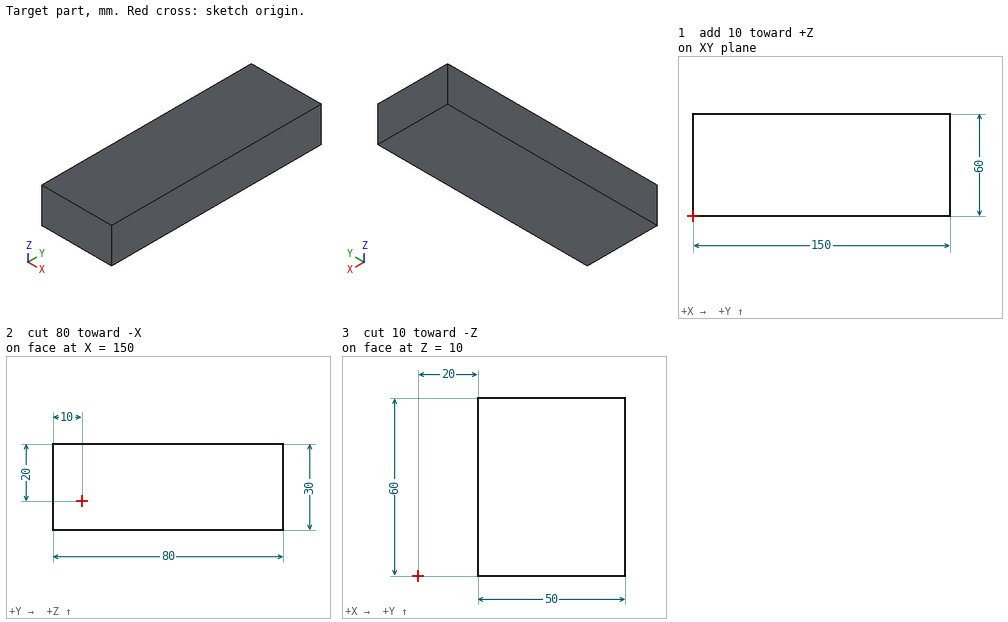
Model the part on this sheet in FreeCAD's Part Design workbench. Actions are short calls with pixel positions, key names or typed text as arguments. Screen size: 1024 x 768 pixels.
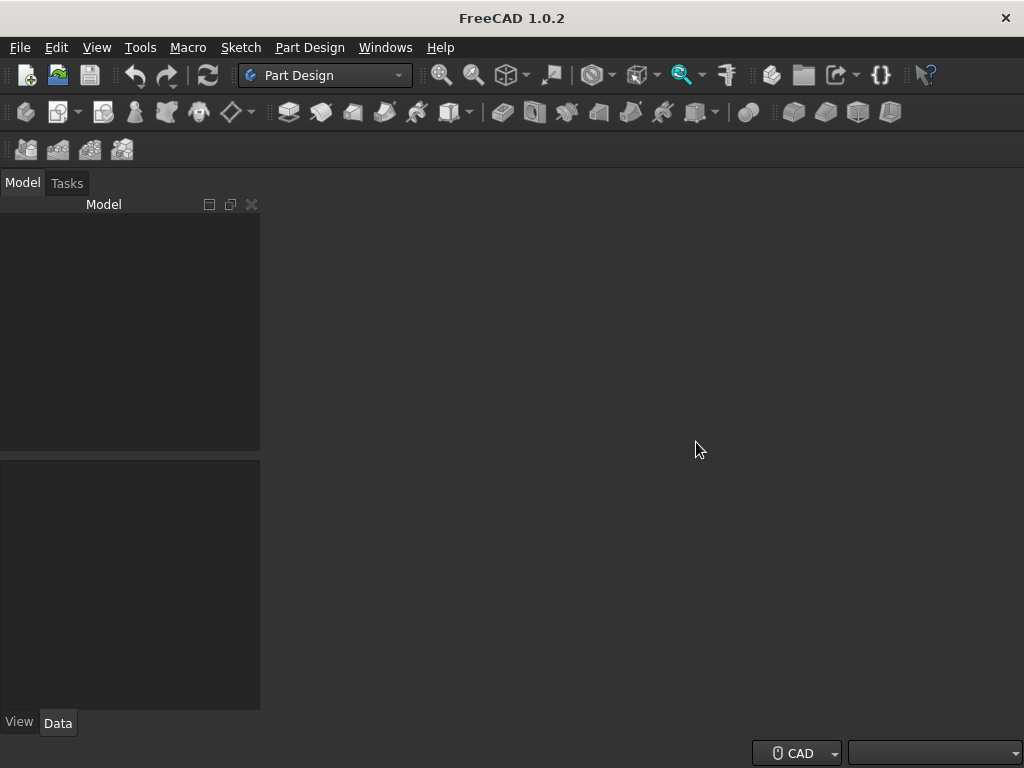
click(26, 76)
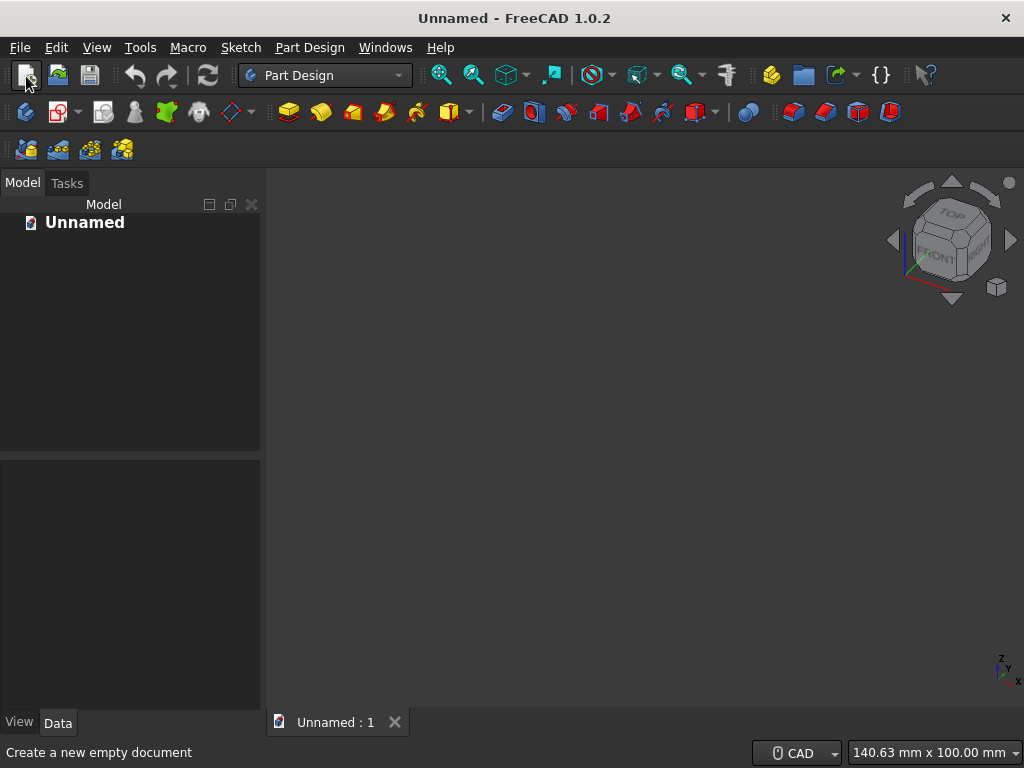
click(58, 112)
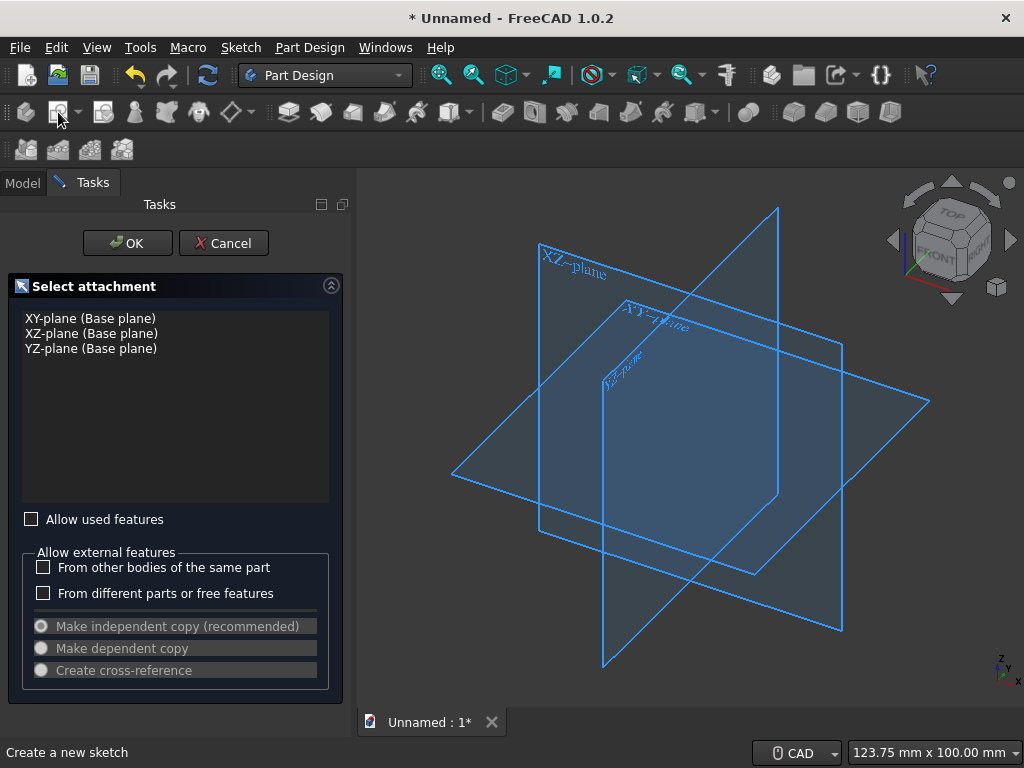
click(82, 318)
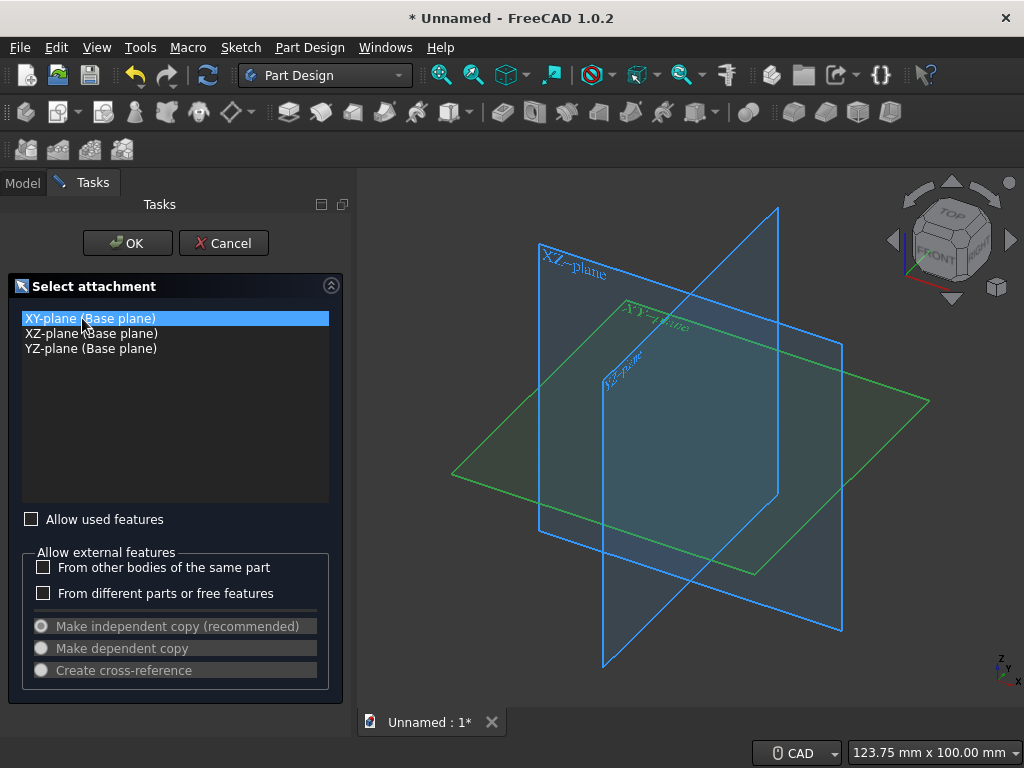
click(128, 243)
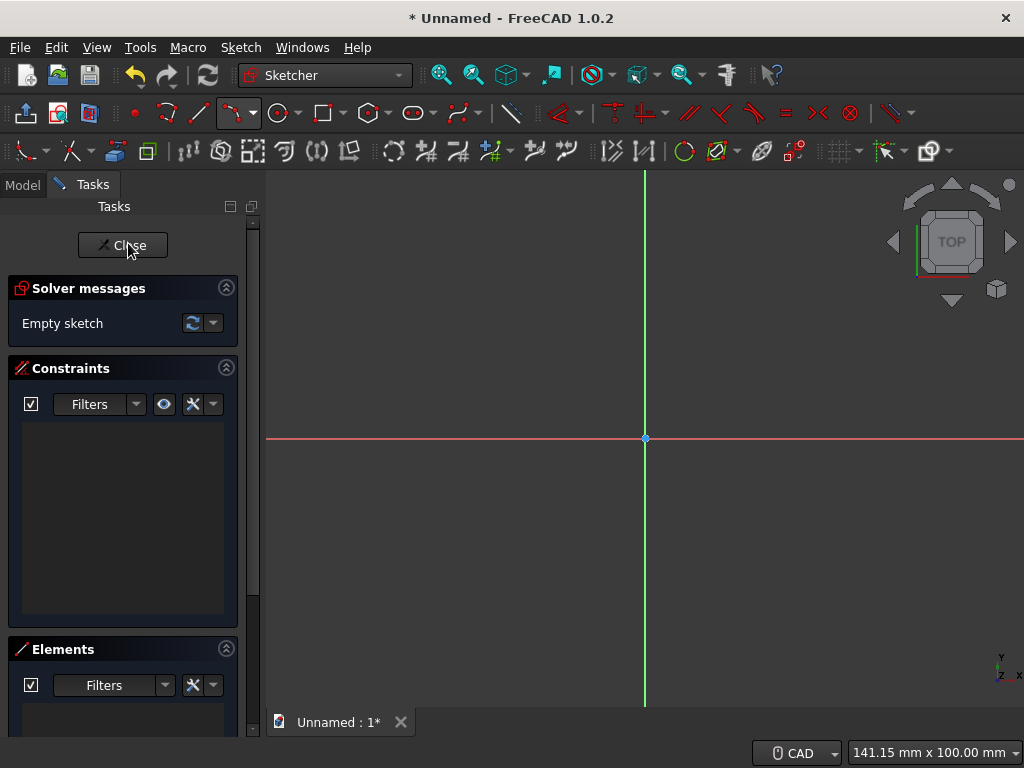
scroll(294, 570, down, 4)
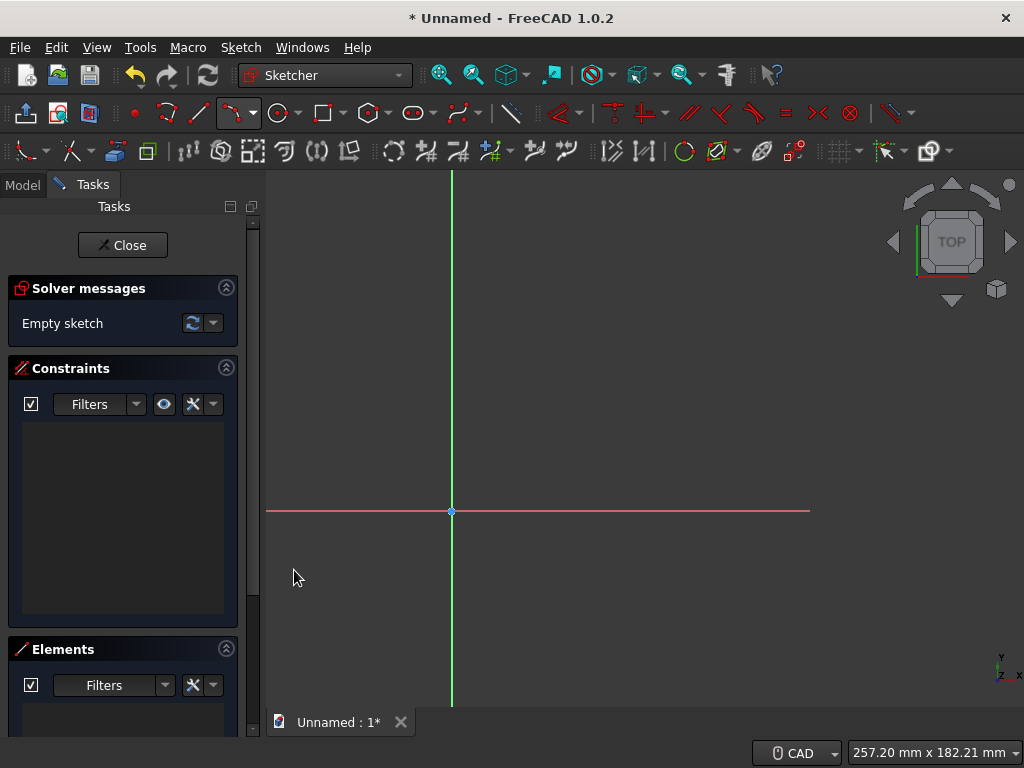
click(324, 114)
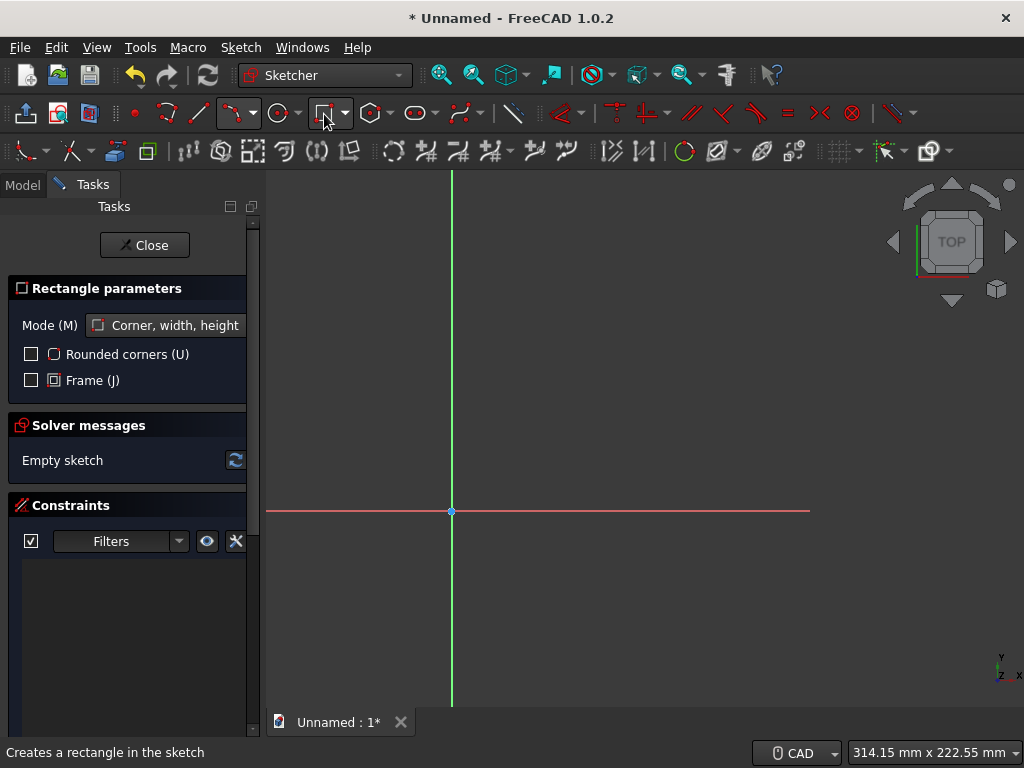
click(452, 511)
move(814, 367)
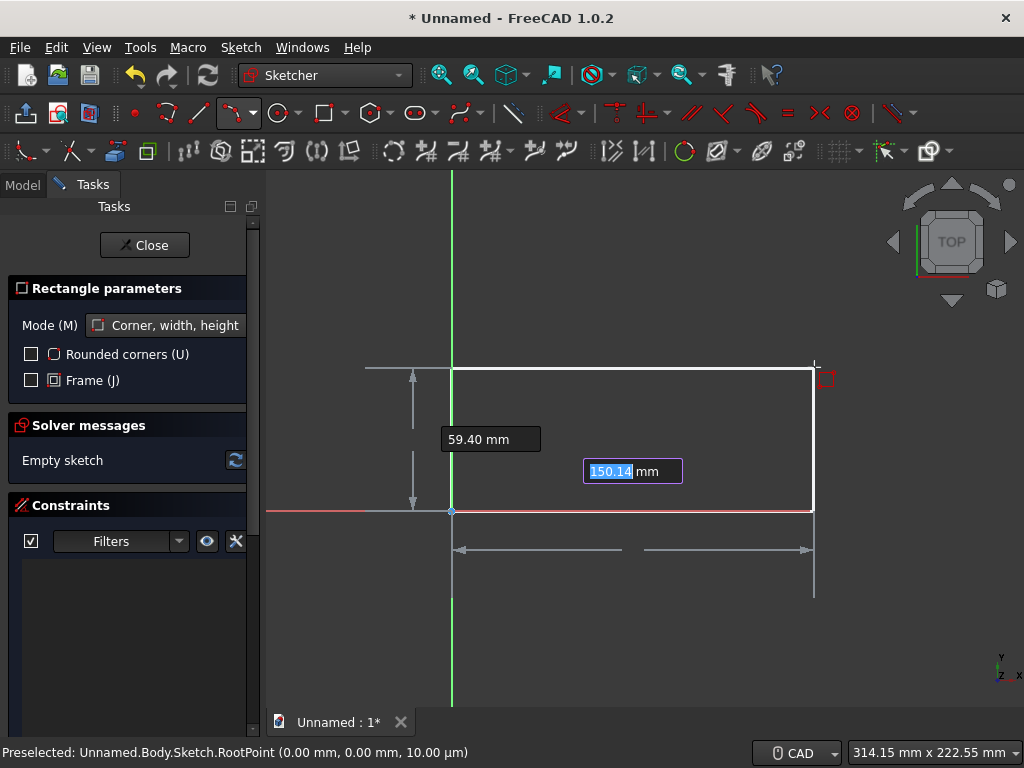
text(150)
key(Tab)
text(60)
key(Return)
key(Escape)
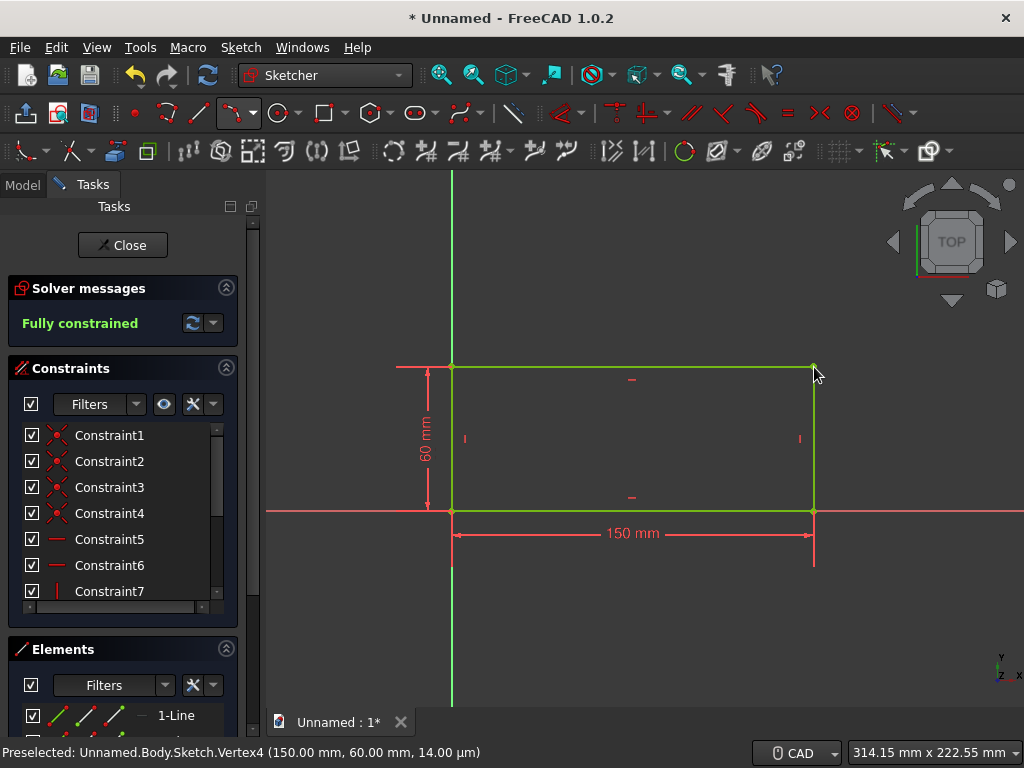
click(123, 245)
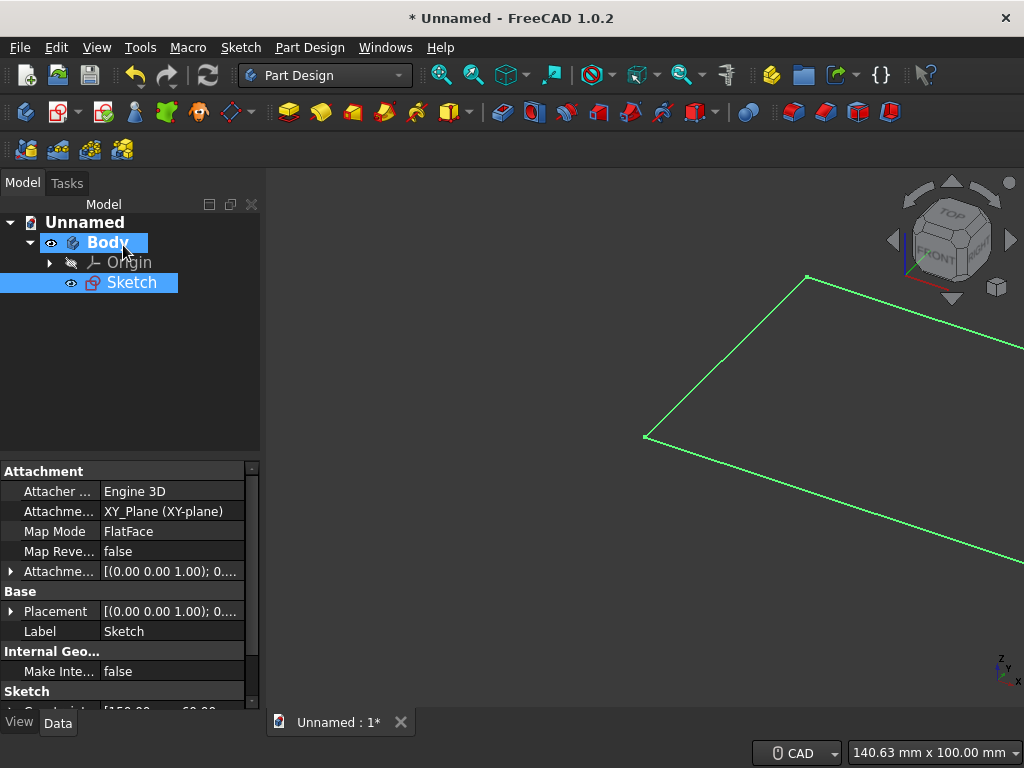
click(290, 112)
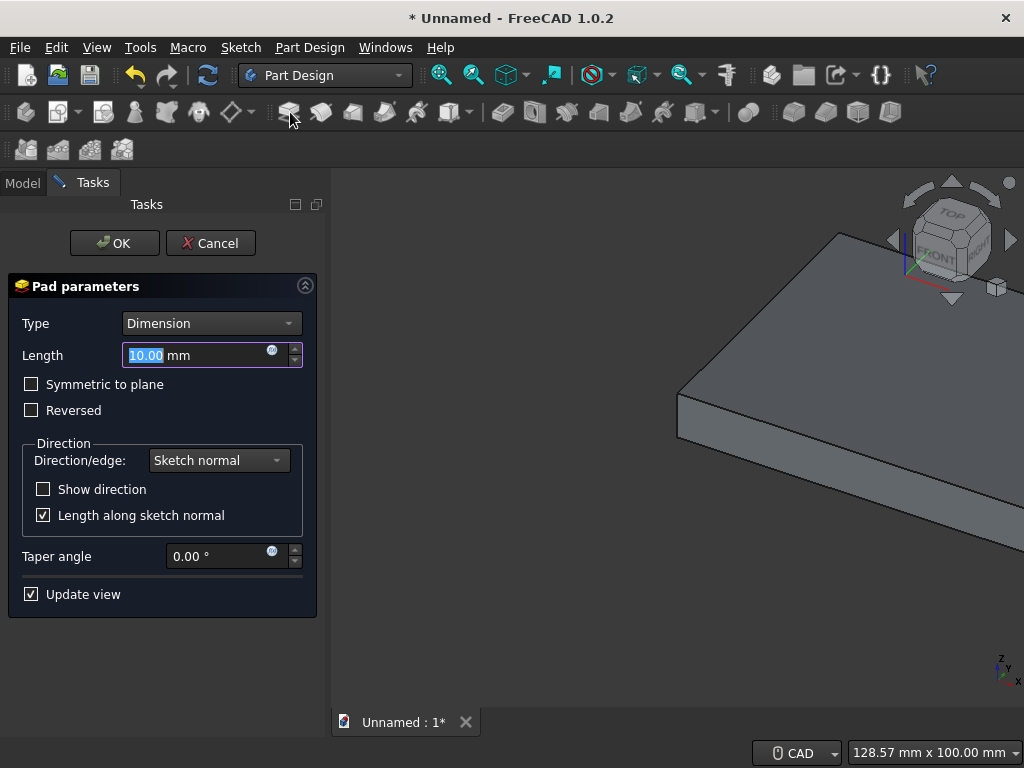
text(10)
key(Tab)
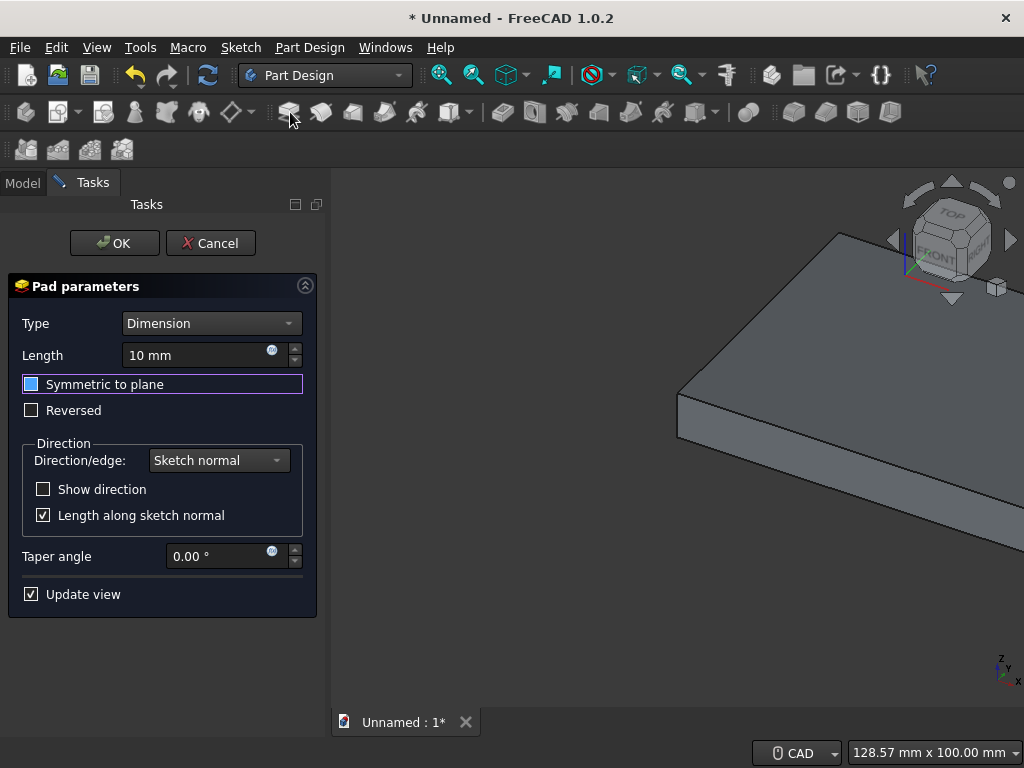
click(115, 243)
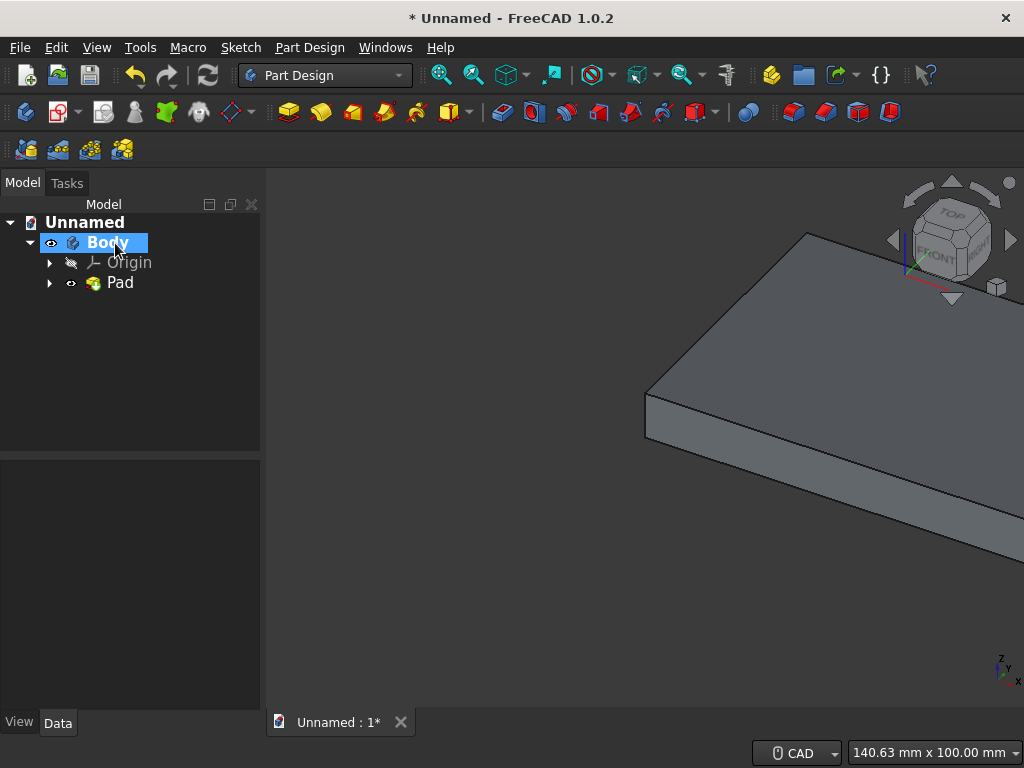
click(442, 76)